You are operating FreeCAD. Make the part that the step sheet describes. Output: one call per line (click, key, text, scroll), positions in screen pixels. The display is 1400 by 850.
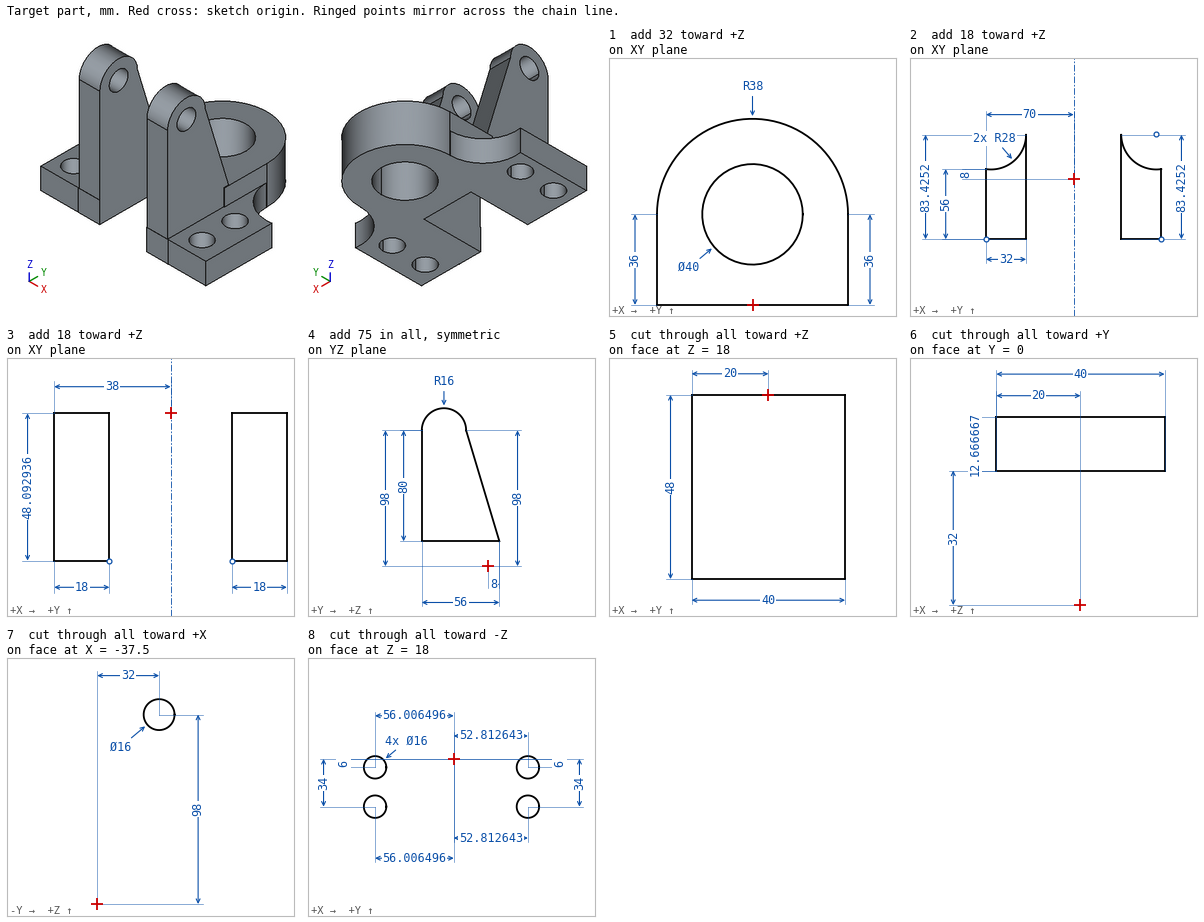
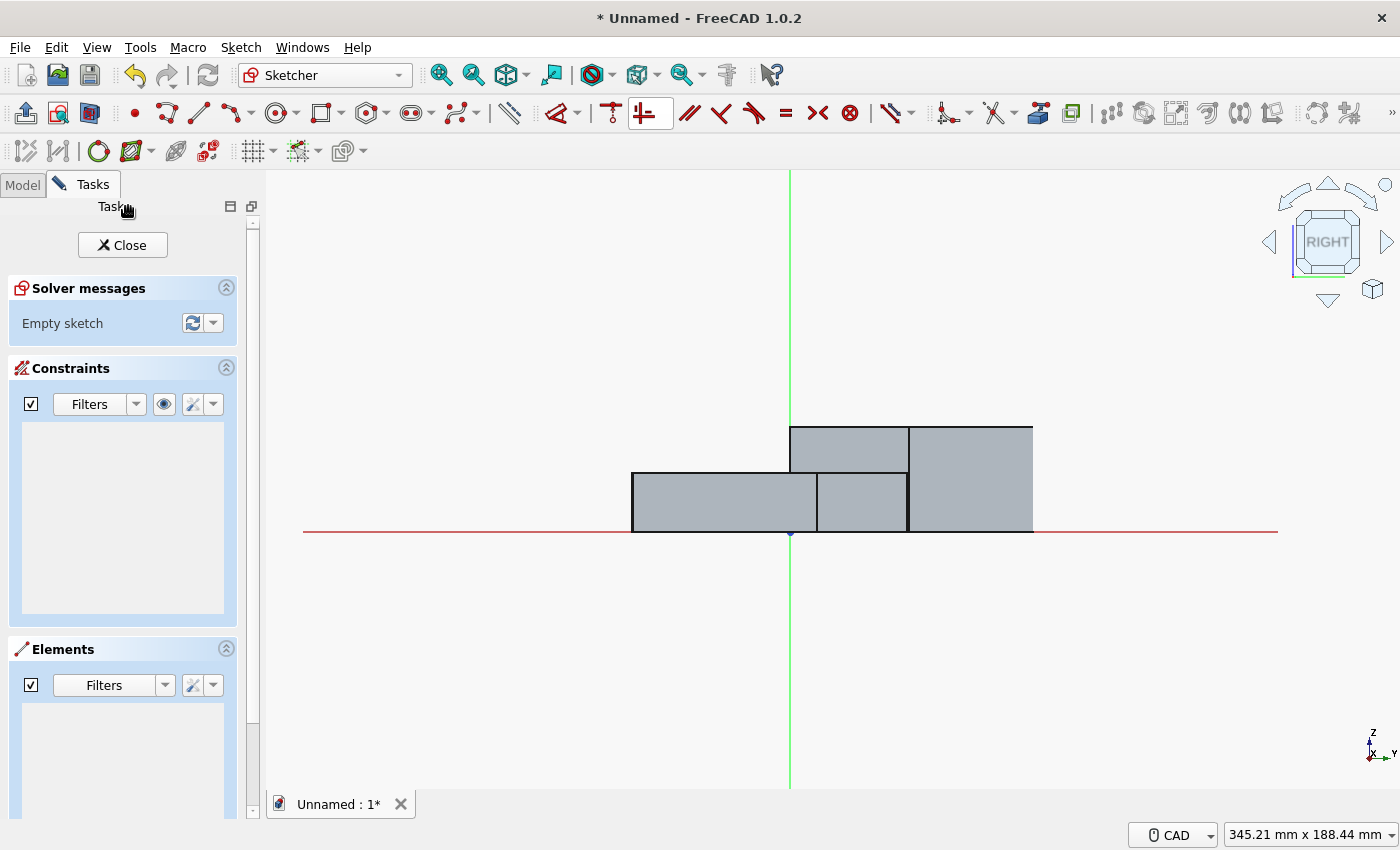
click(90, 114)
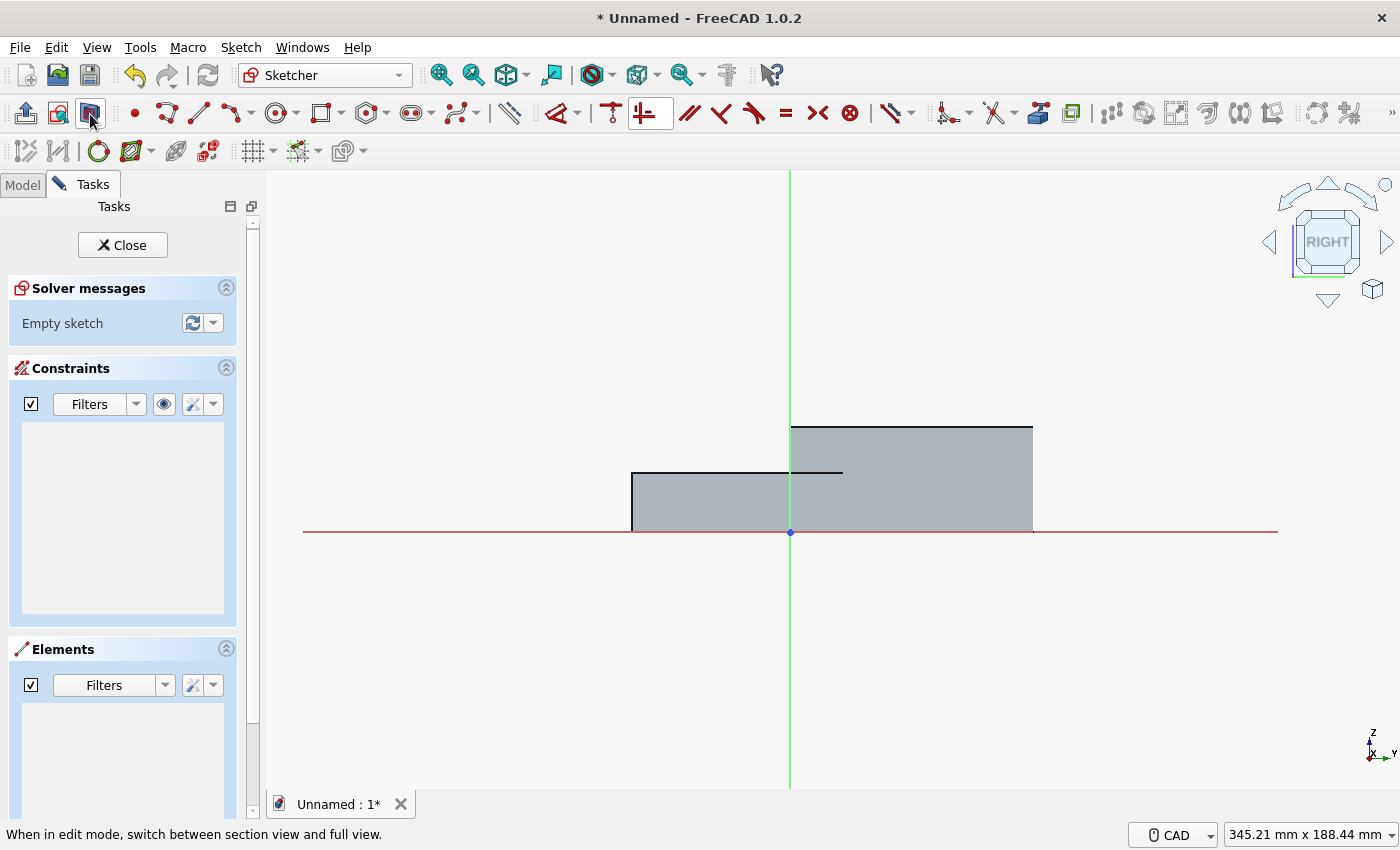
scroll(944, 761, down, 1)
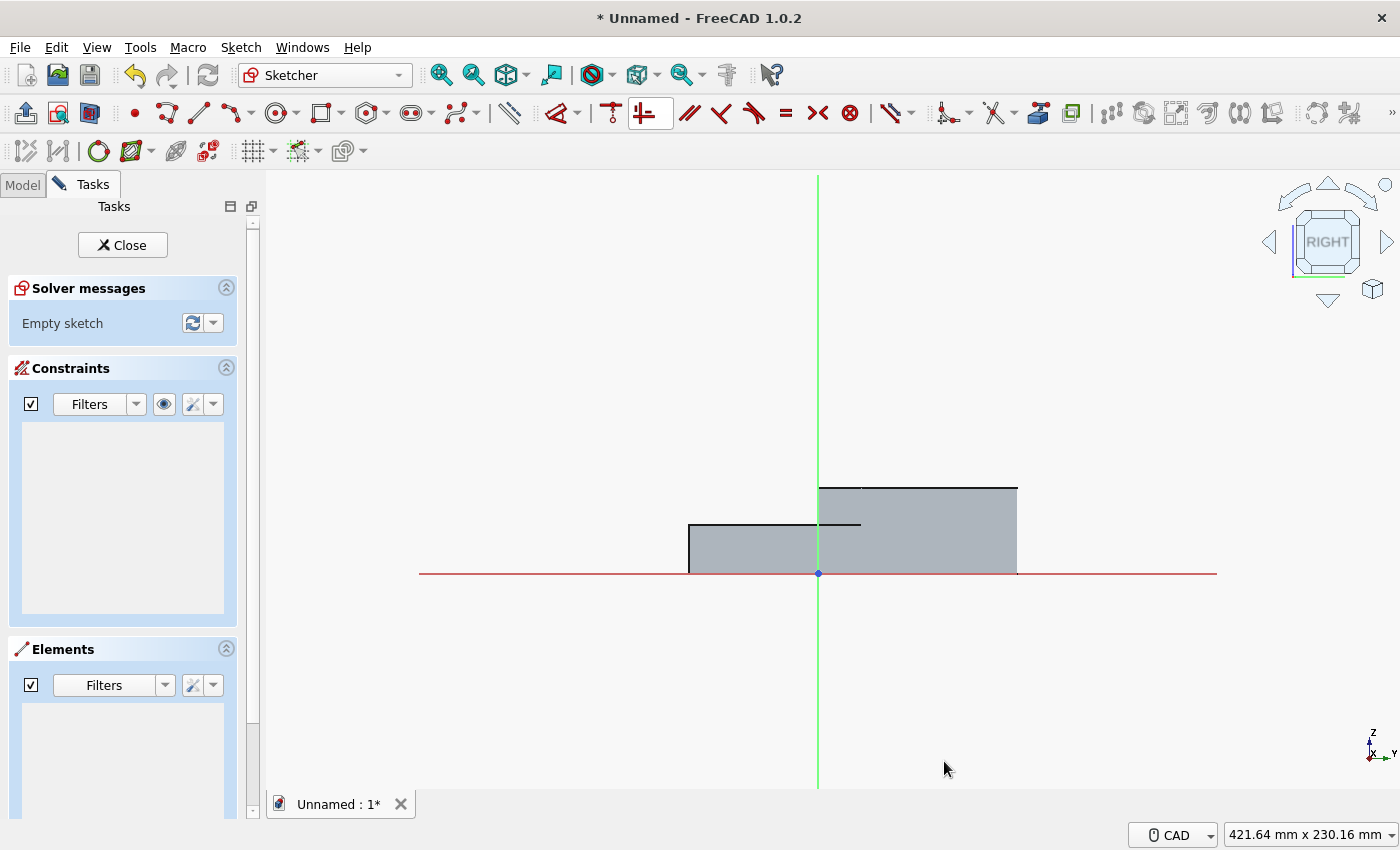
click(168, 114)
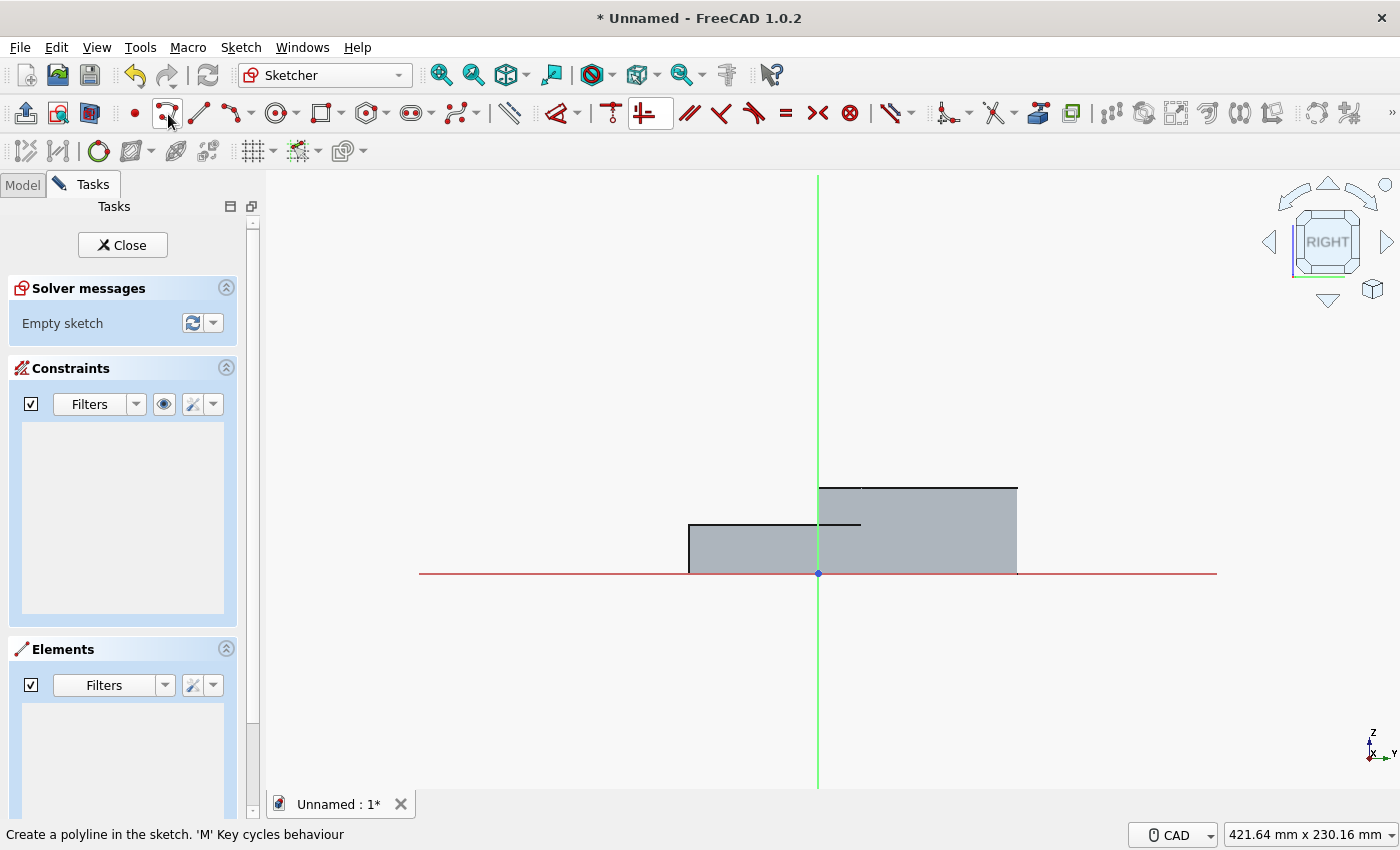
click(689, 310)
click(689, 525)
click(840, 525)
click(775, 310)
right_click(775, 310)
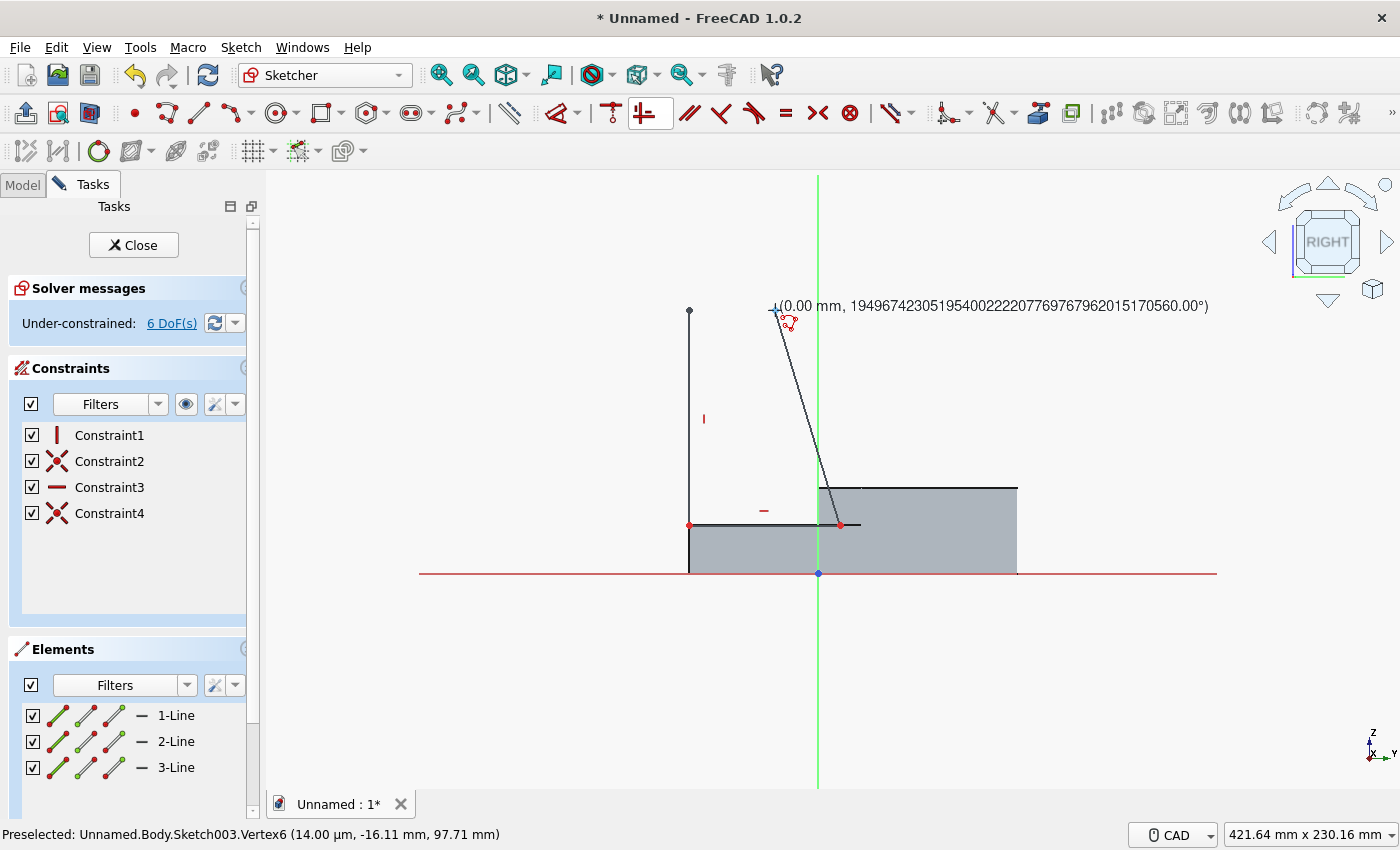
click(232, 114)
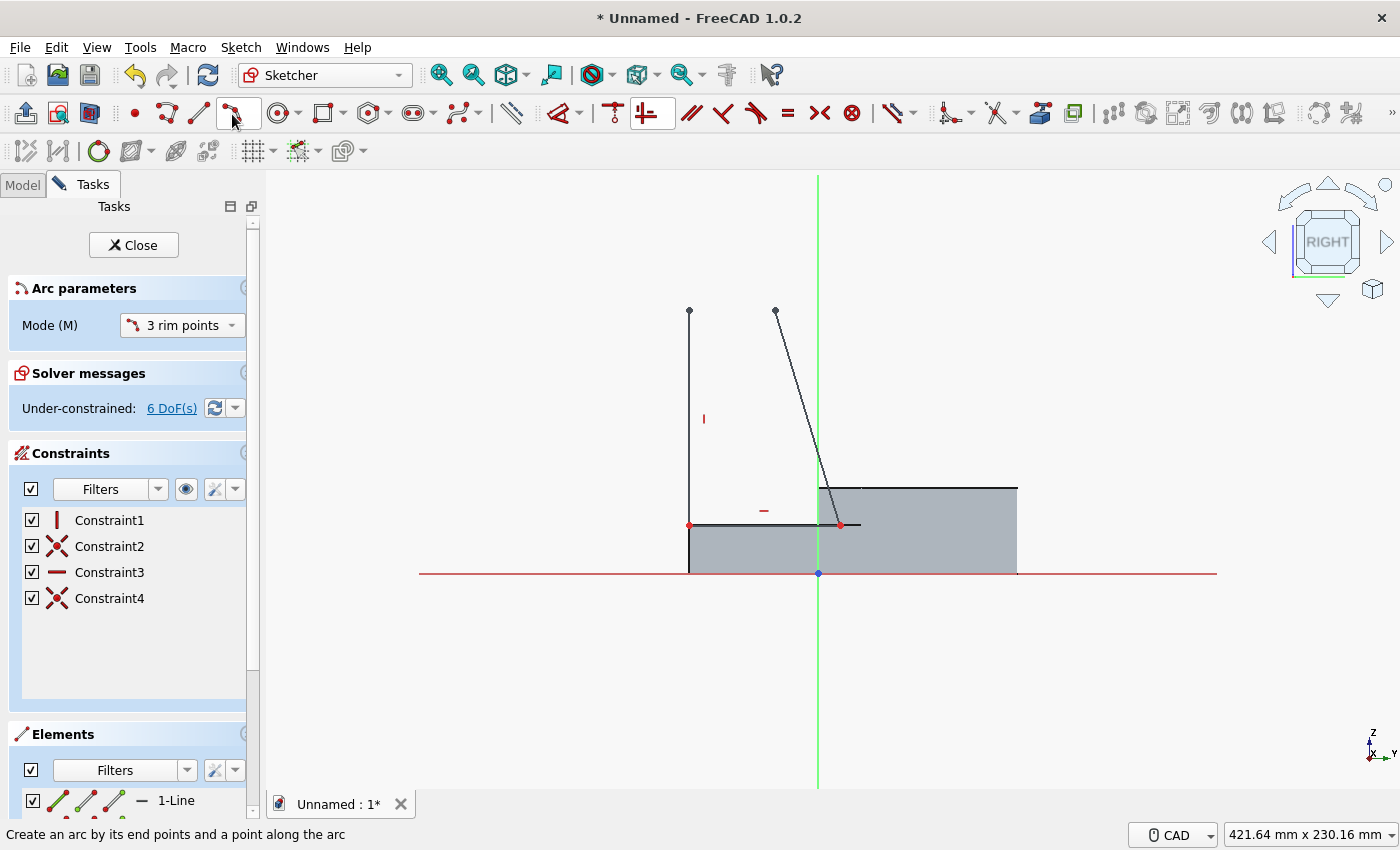
click(775, 311)
click(689, 311)
click(732, 267)
key(Escape)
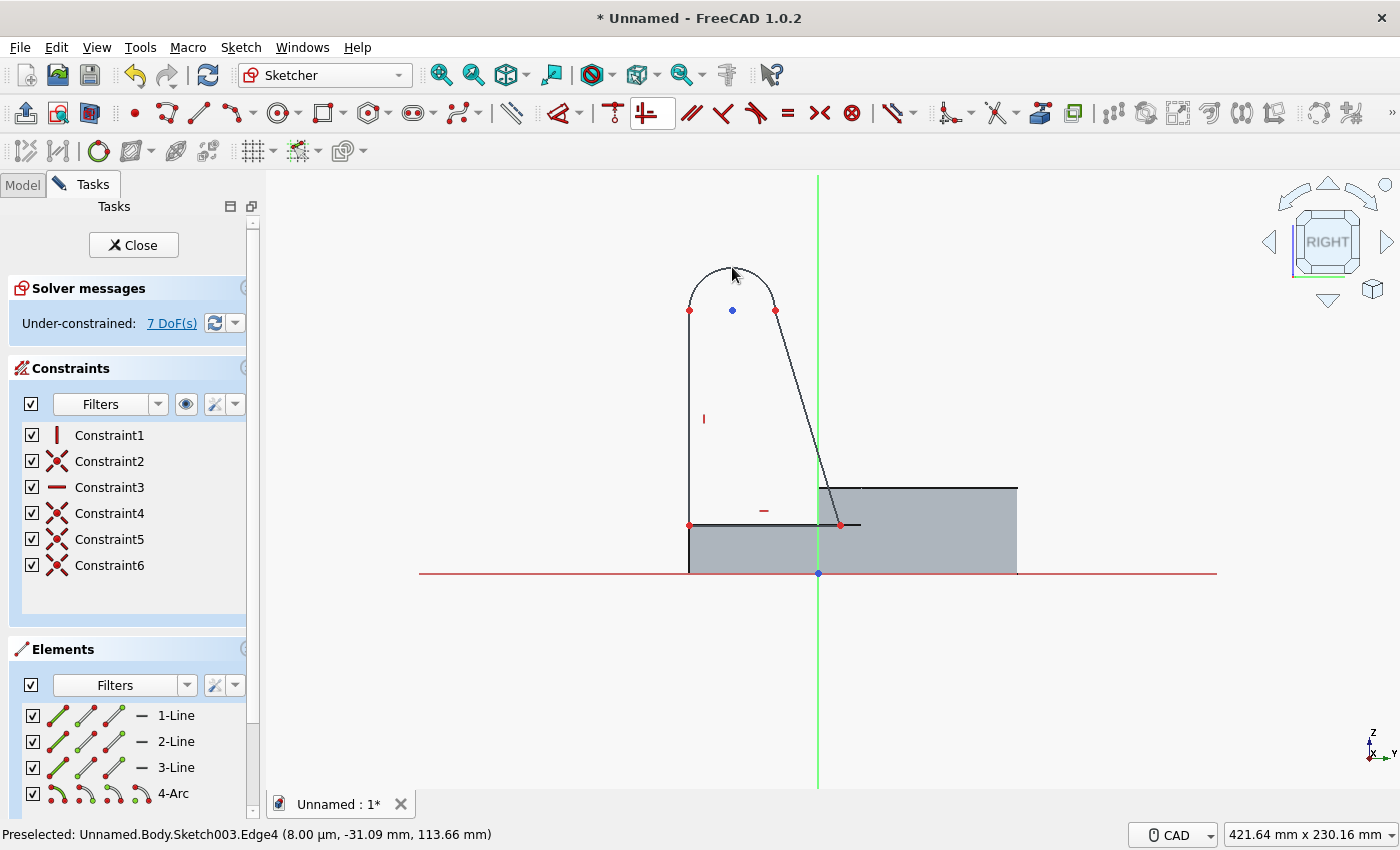
click(689, 376)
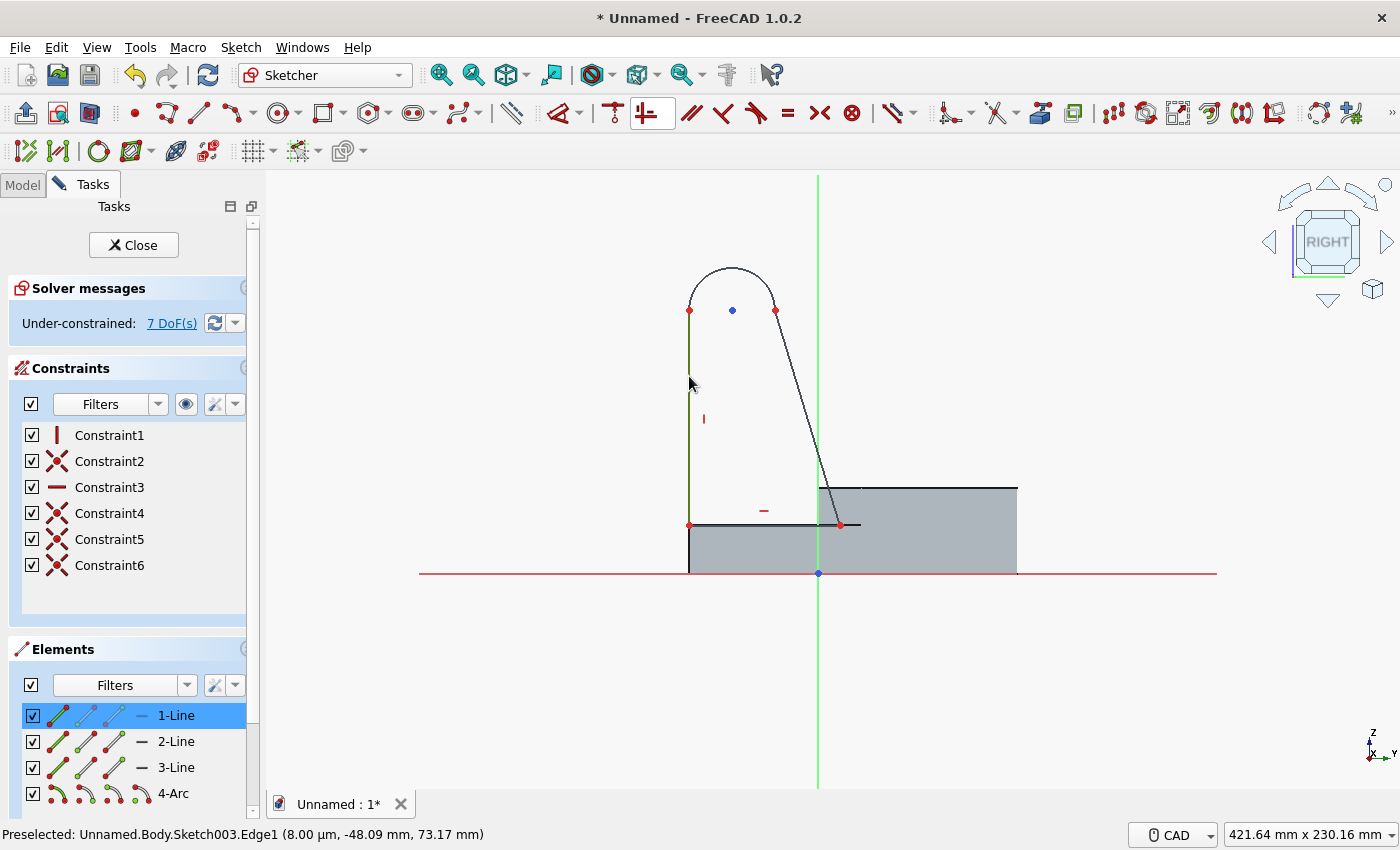
click(757, 276)